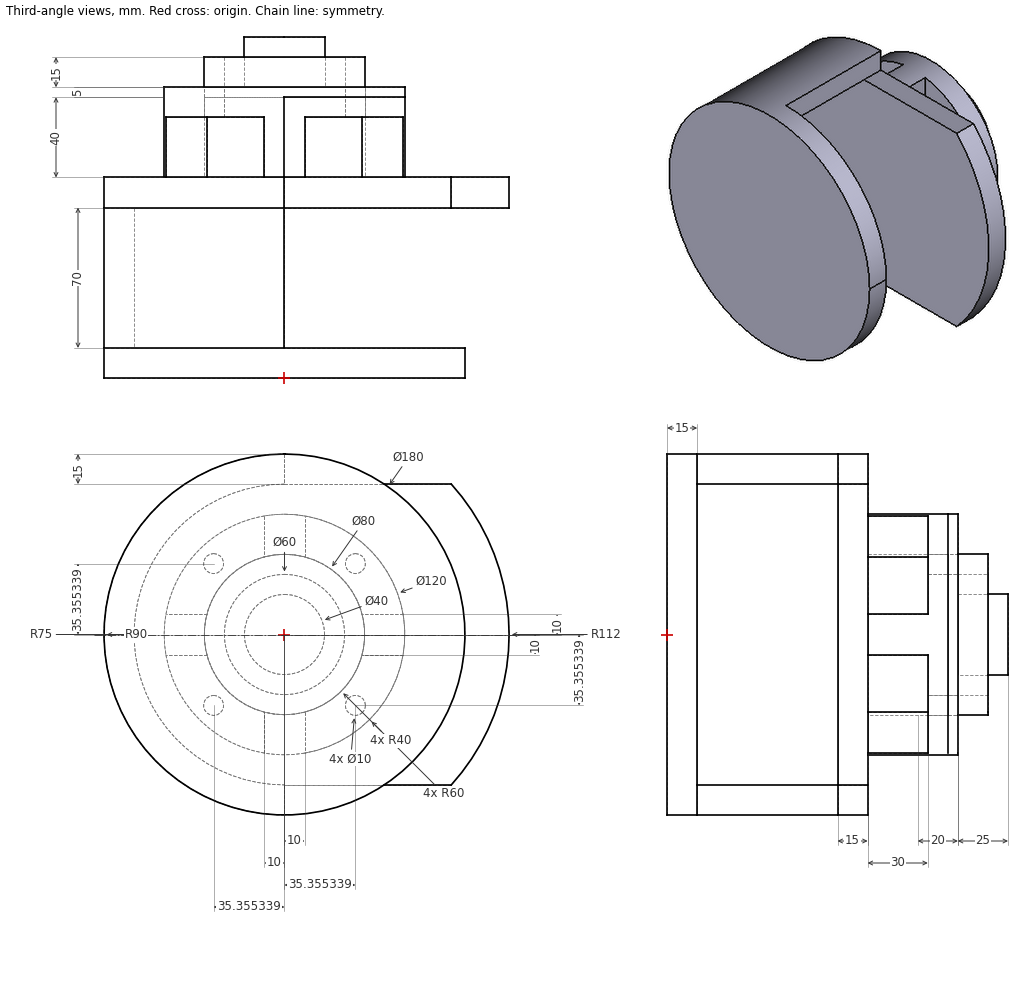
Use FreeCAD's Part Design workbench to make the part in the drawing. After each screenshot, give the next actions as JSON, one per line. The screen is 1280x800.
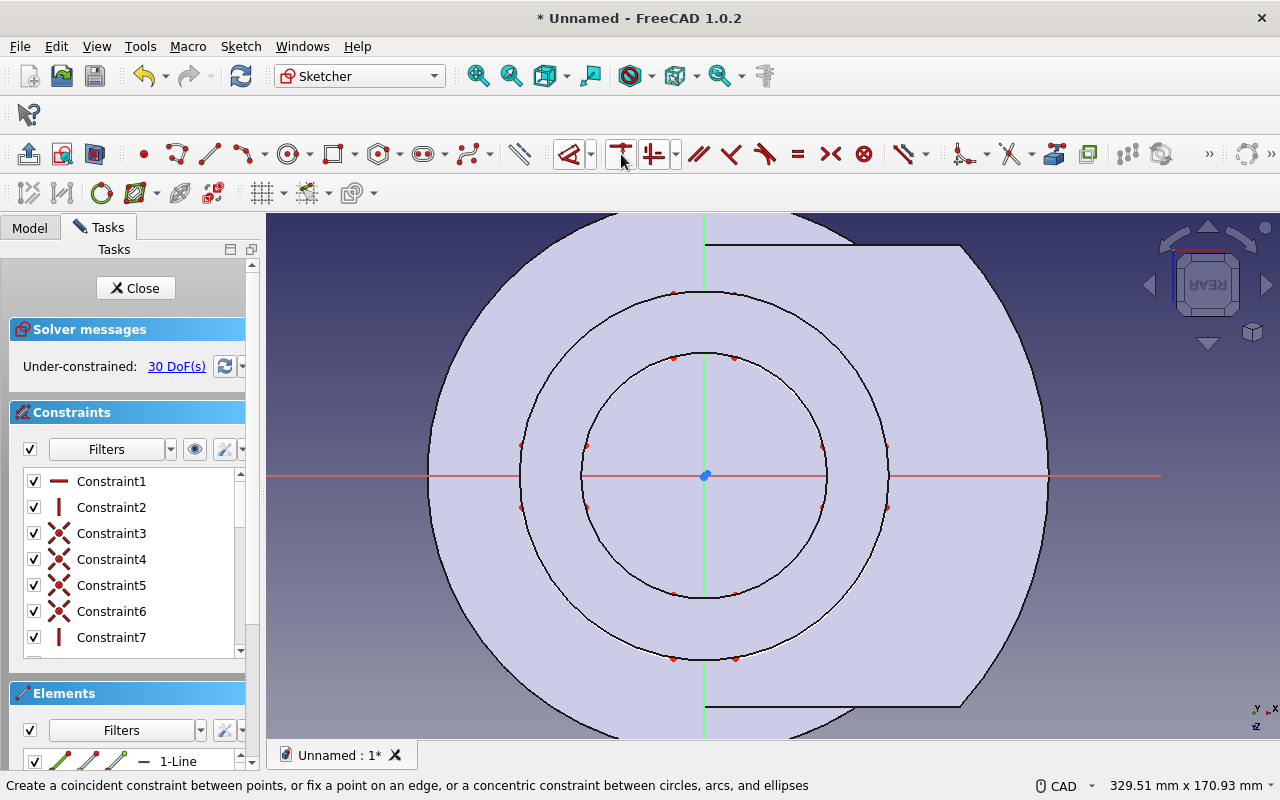
{"action": "left_click", "coordinate": [863, 382]}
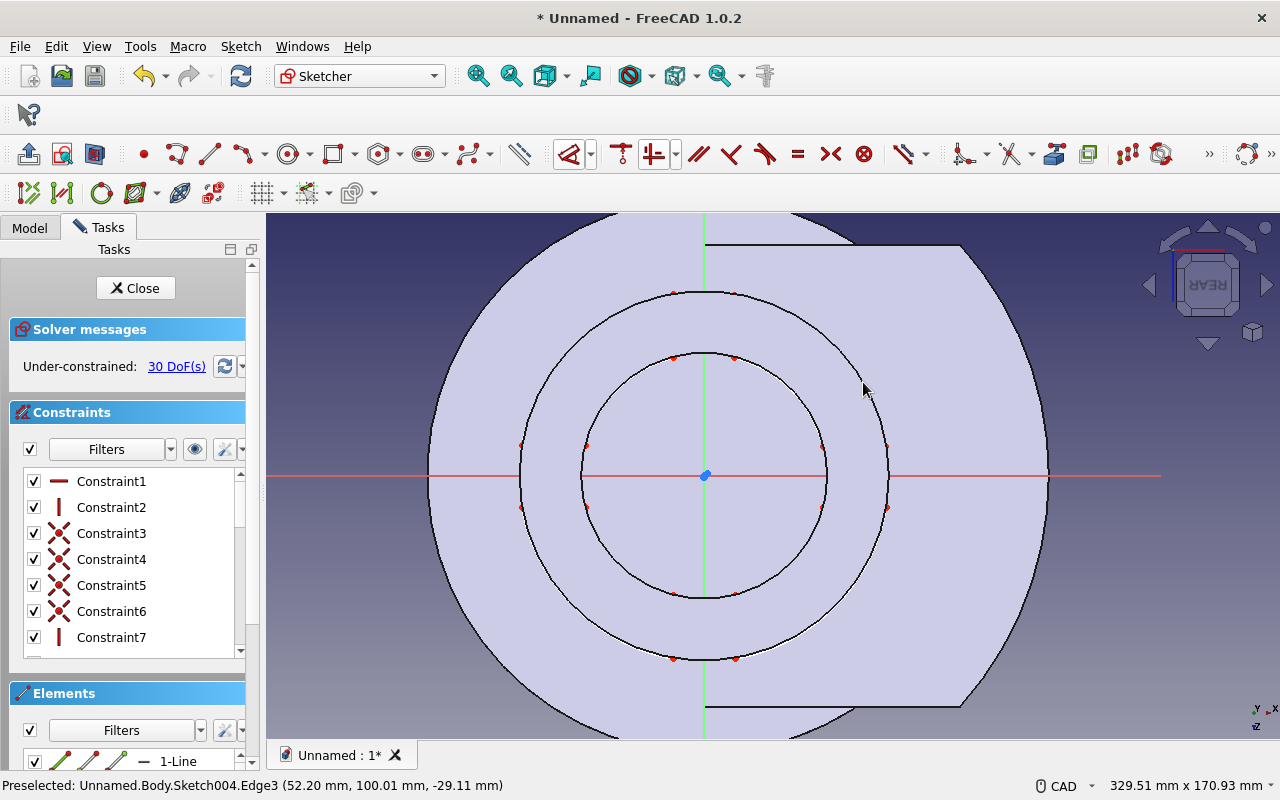
{"action": "left_click", "coordinate": [609, 319]}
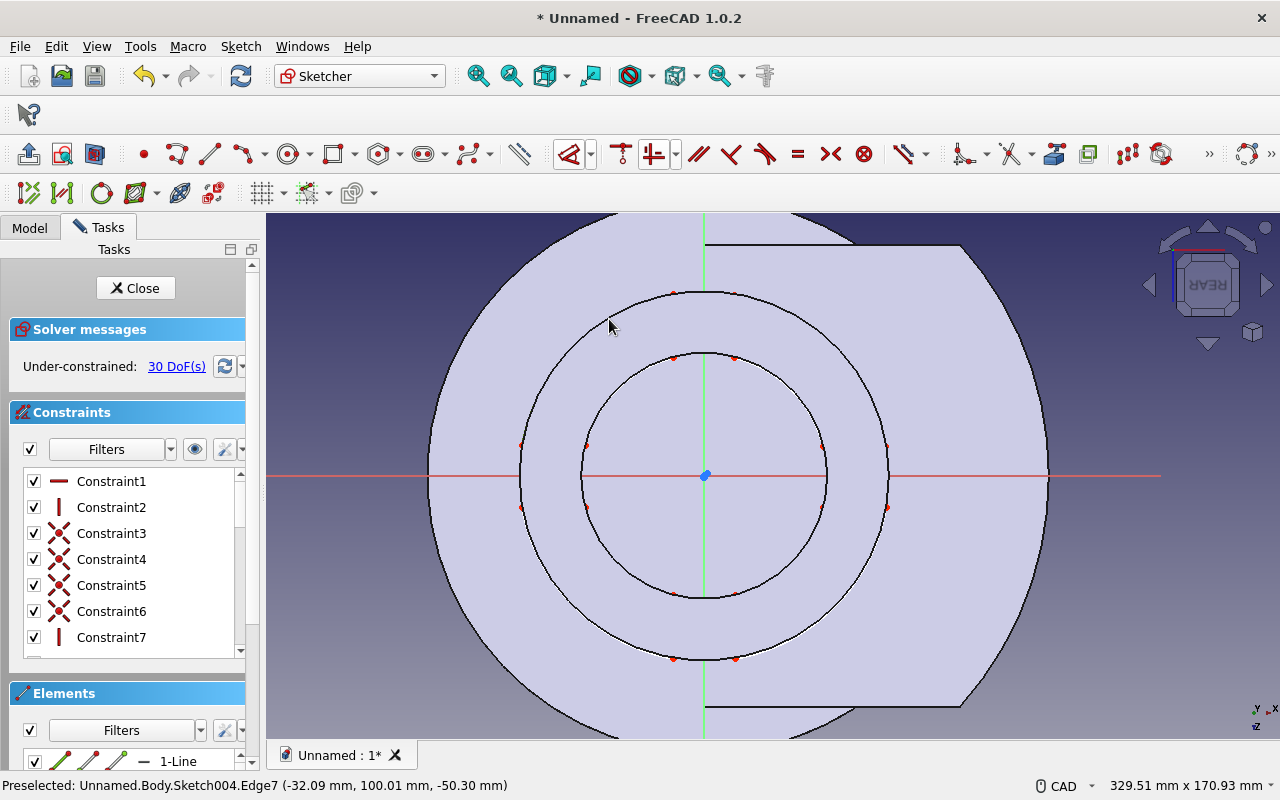
{"action": "left_click", "coordinate": [621, 154]}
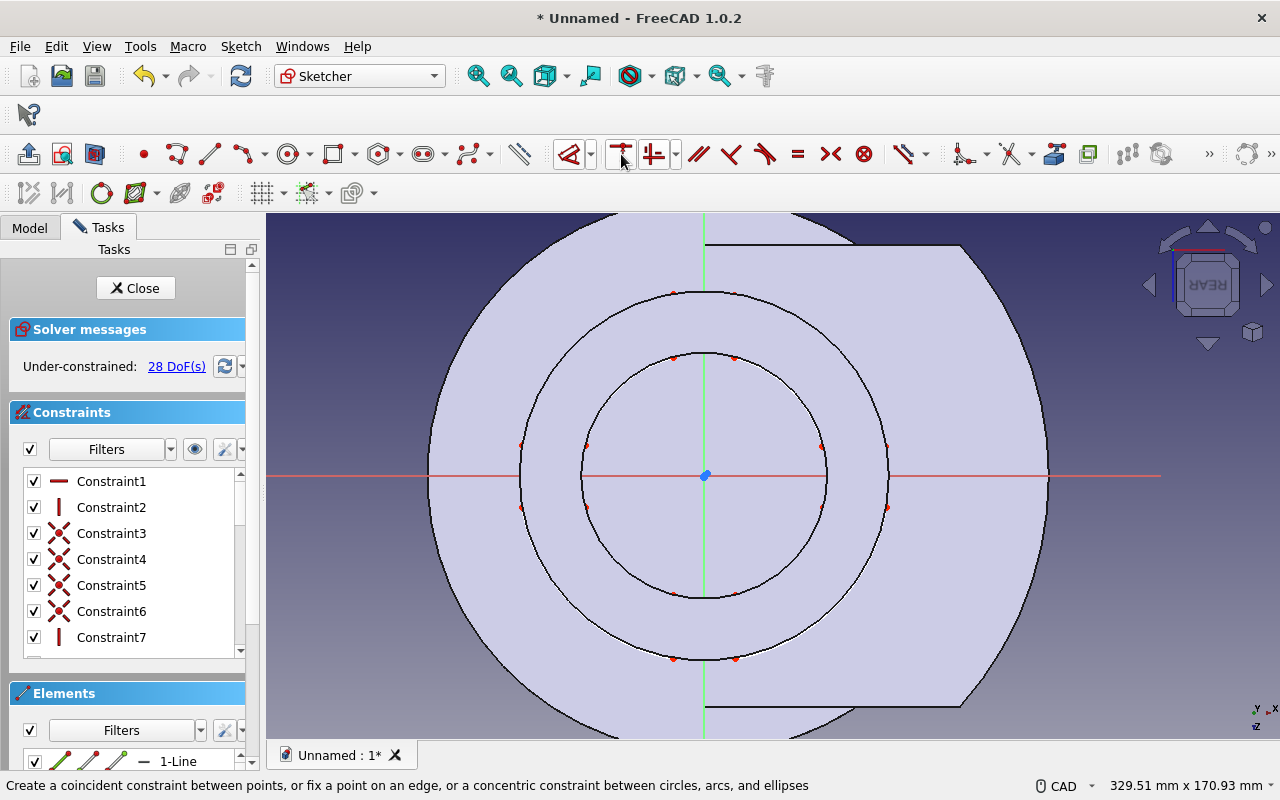
{"action": "left_click", "coordinate": [862, 382]}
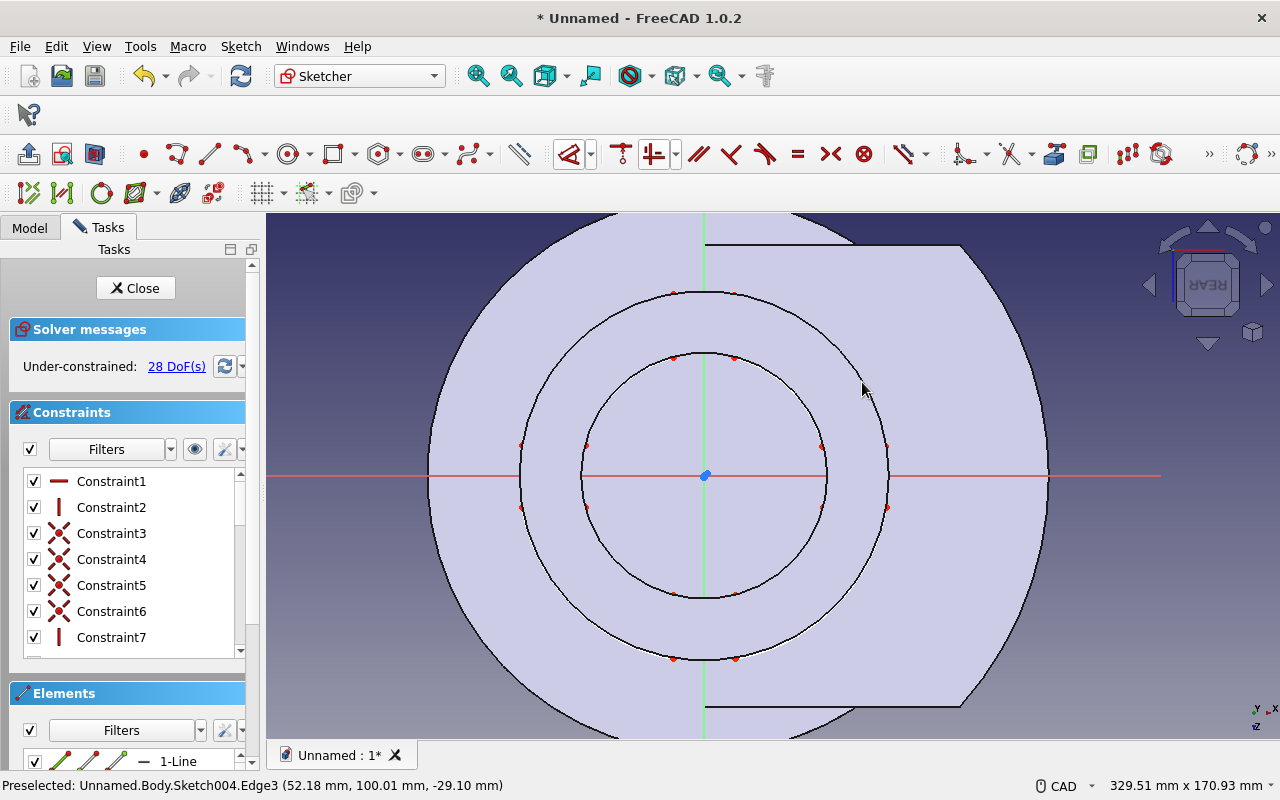
{"action": "left_click", "coordinate": [637, 374]}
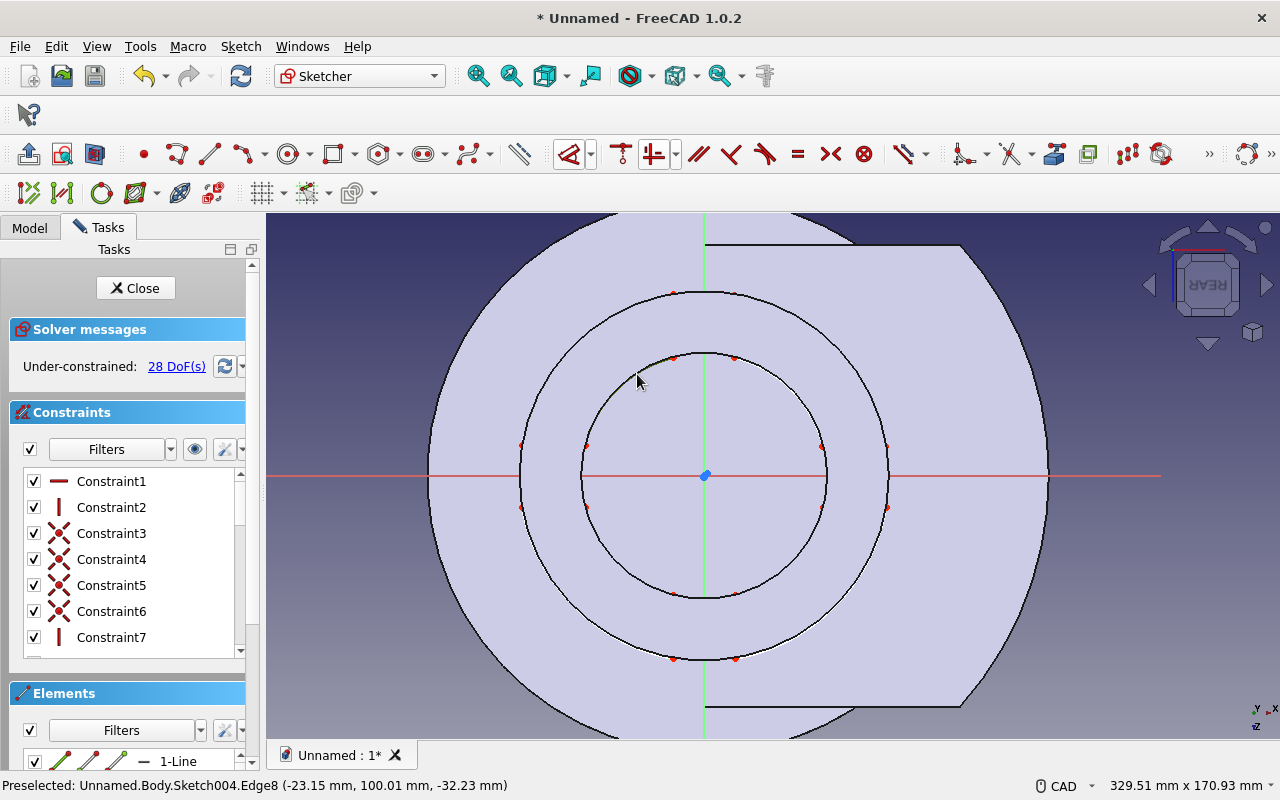
{"action": "key", "text": "c"}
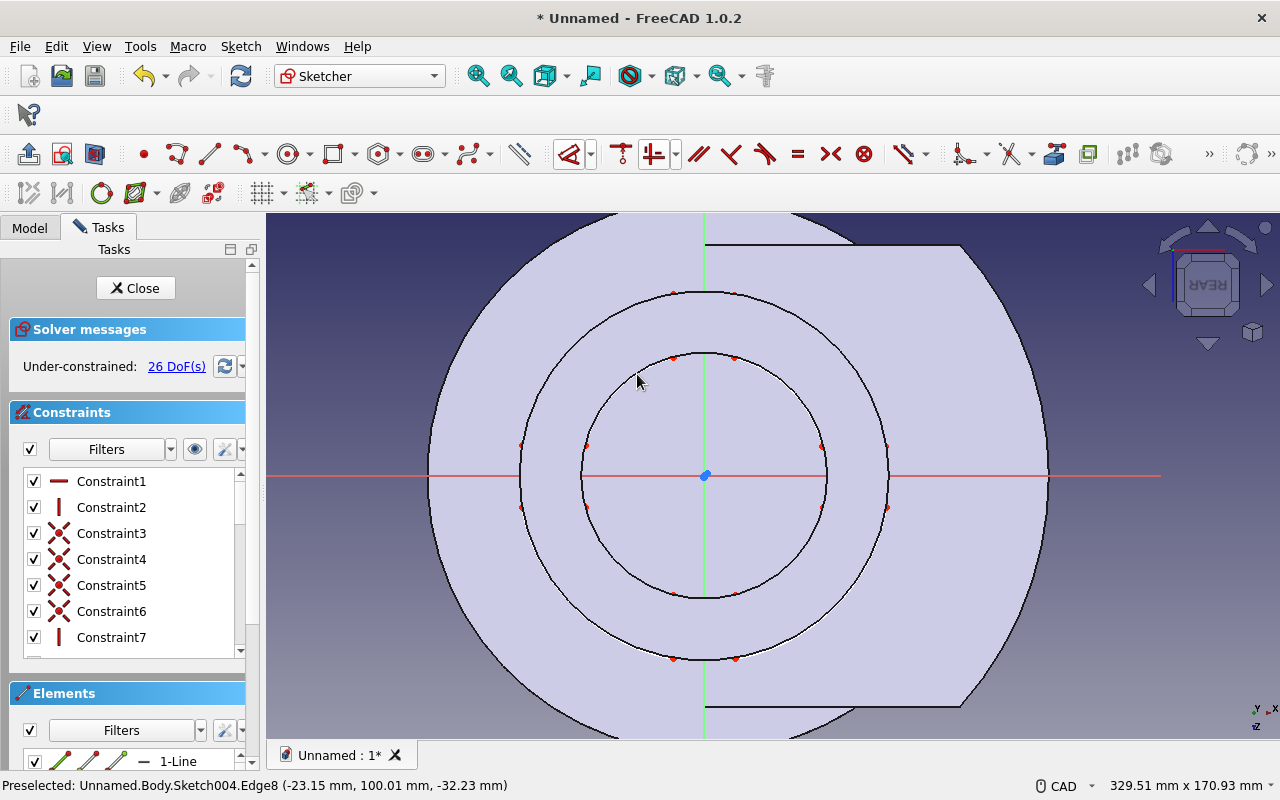
{"action": "left_click", "coordinate": [862, 382]}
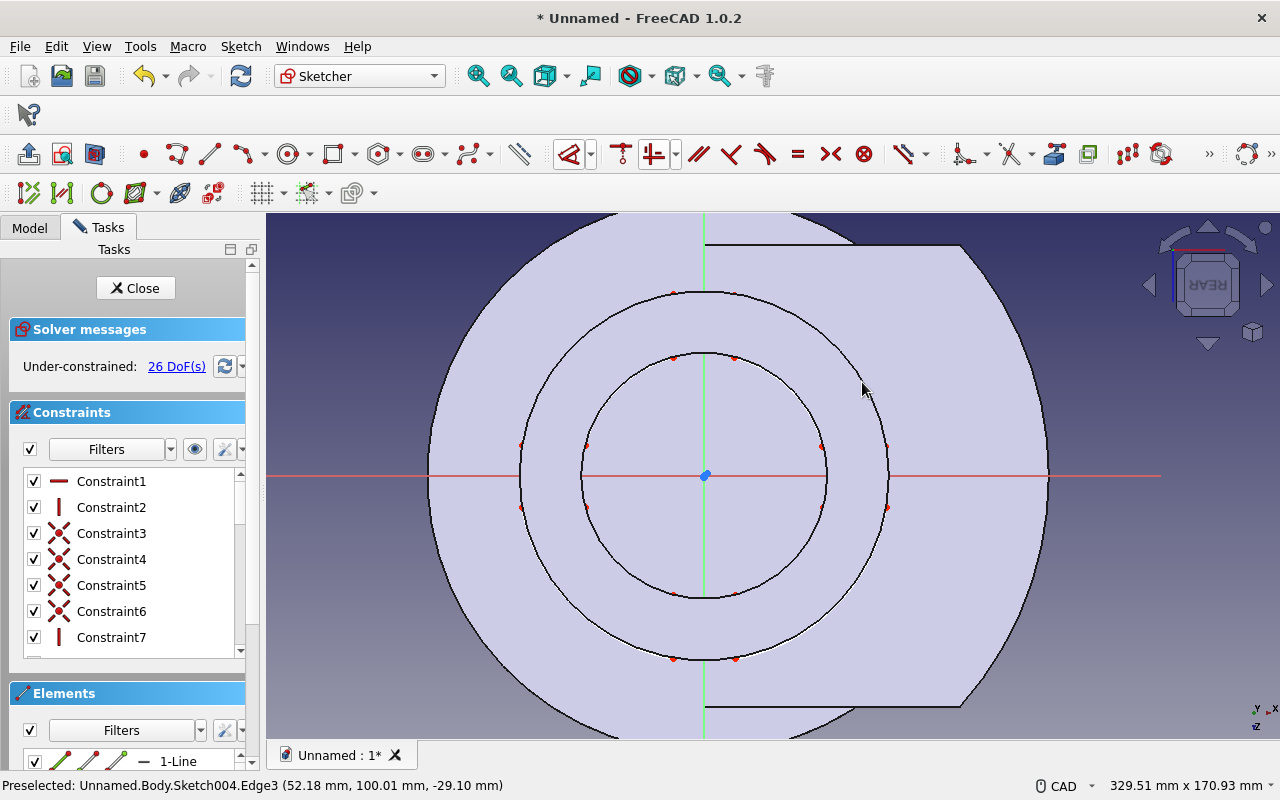
{"action": "left_click", "coordinate": [771, 580]}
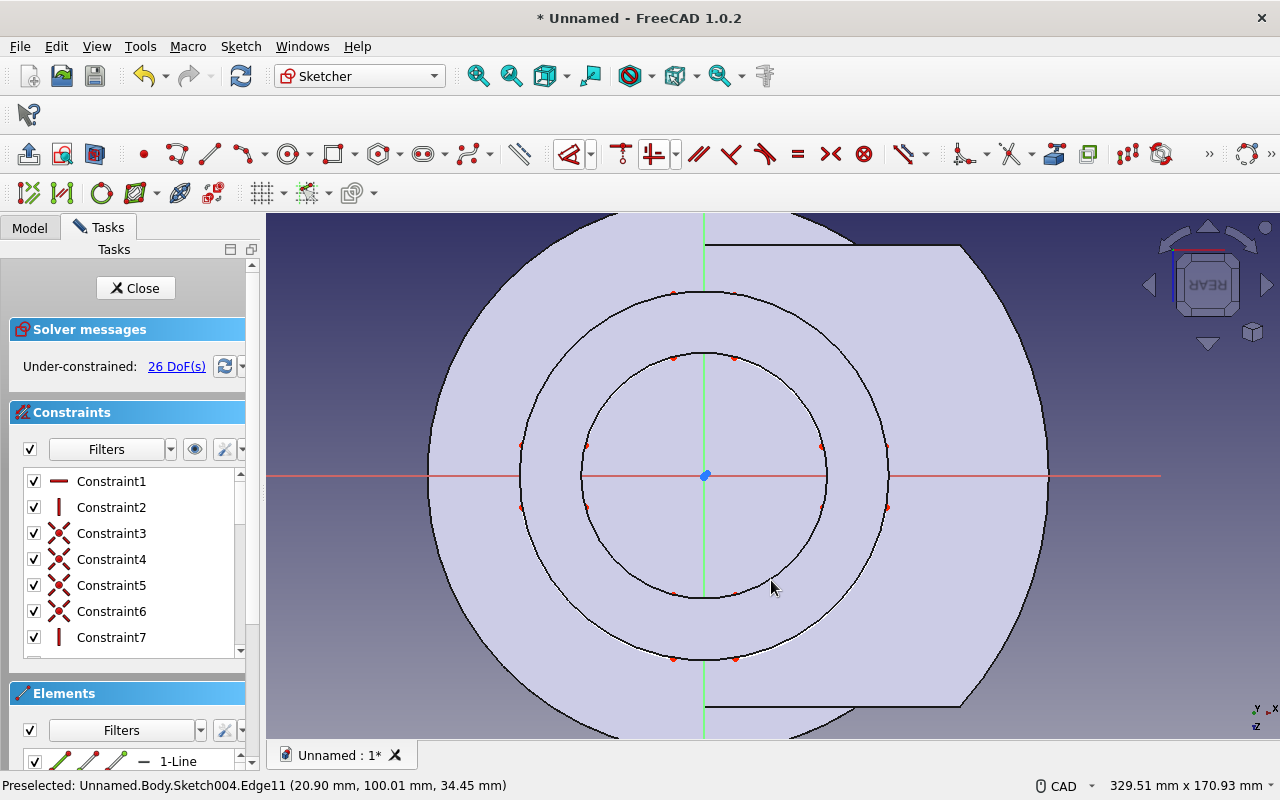
{"action": "key", "text": "c"}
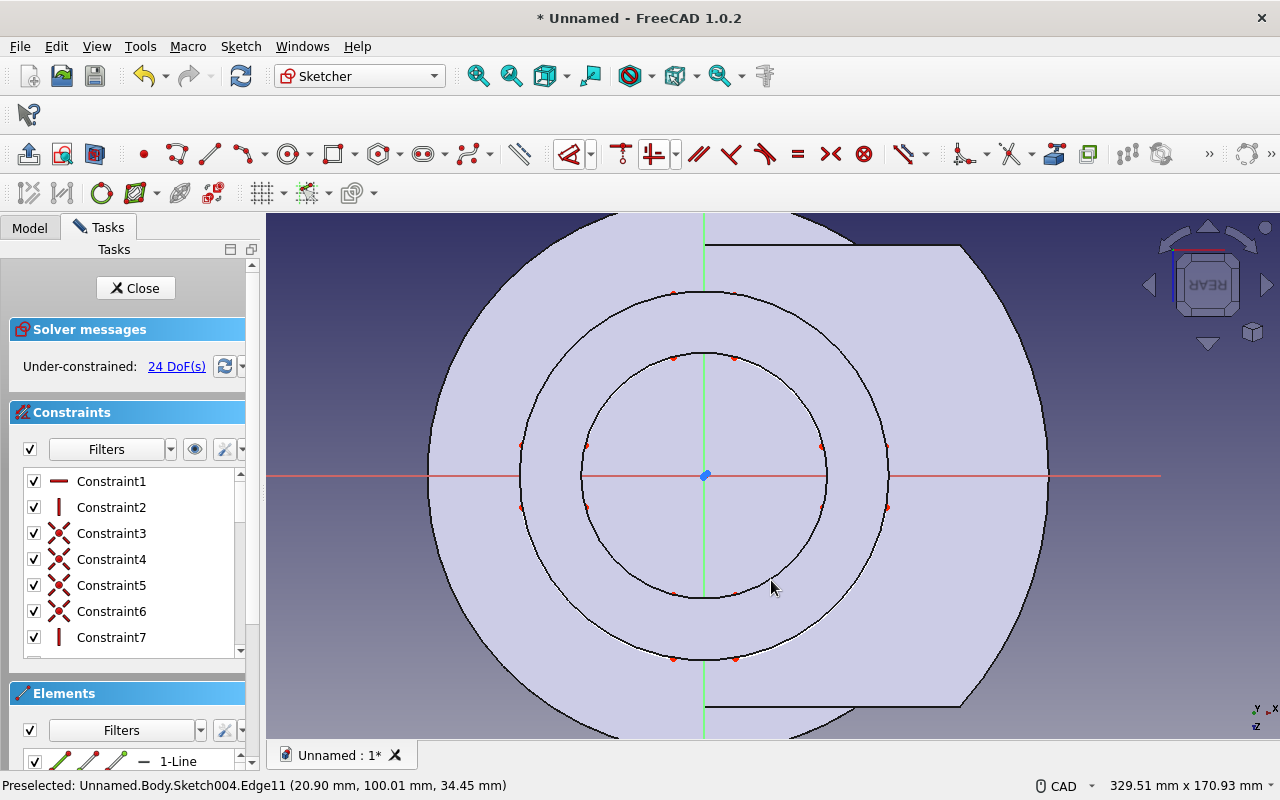
{"action": "left_click", "coordinate": [862, 382]}